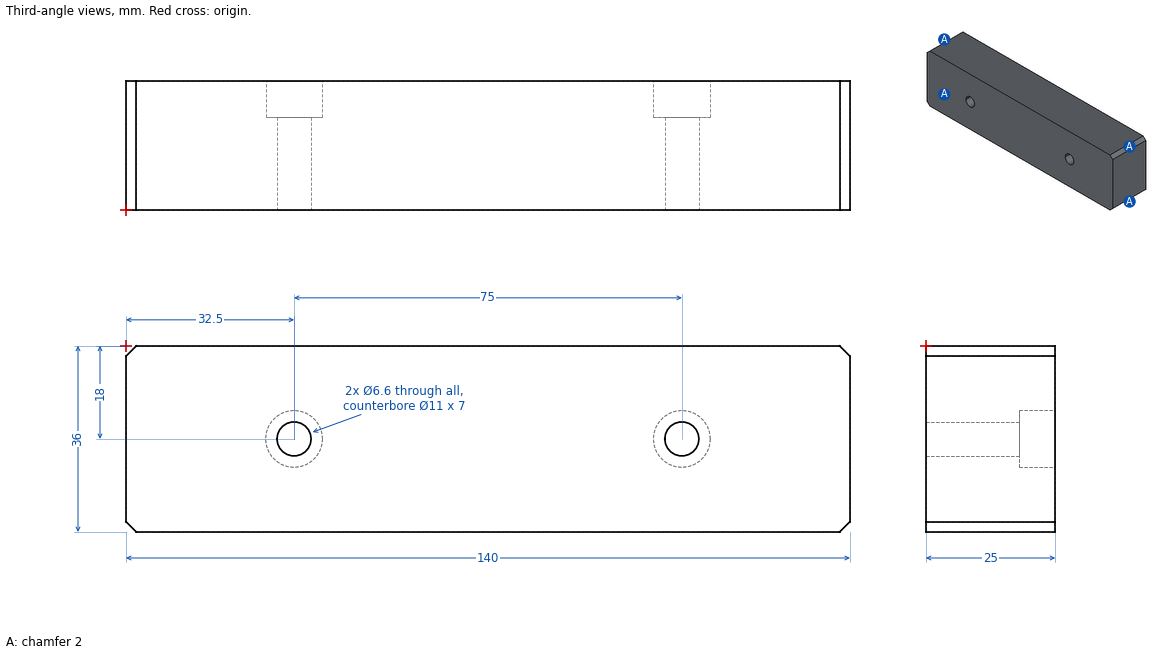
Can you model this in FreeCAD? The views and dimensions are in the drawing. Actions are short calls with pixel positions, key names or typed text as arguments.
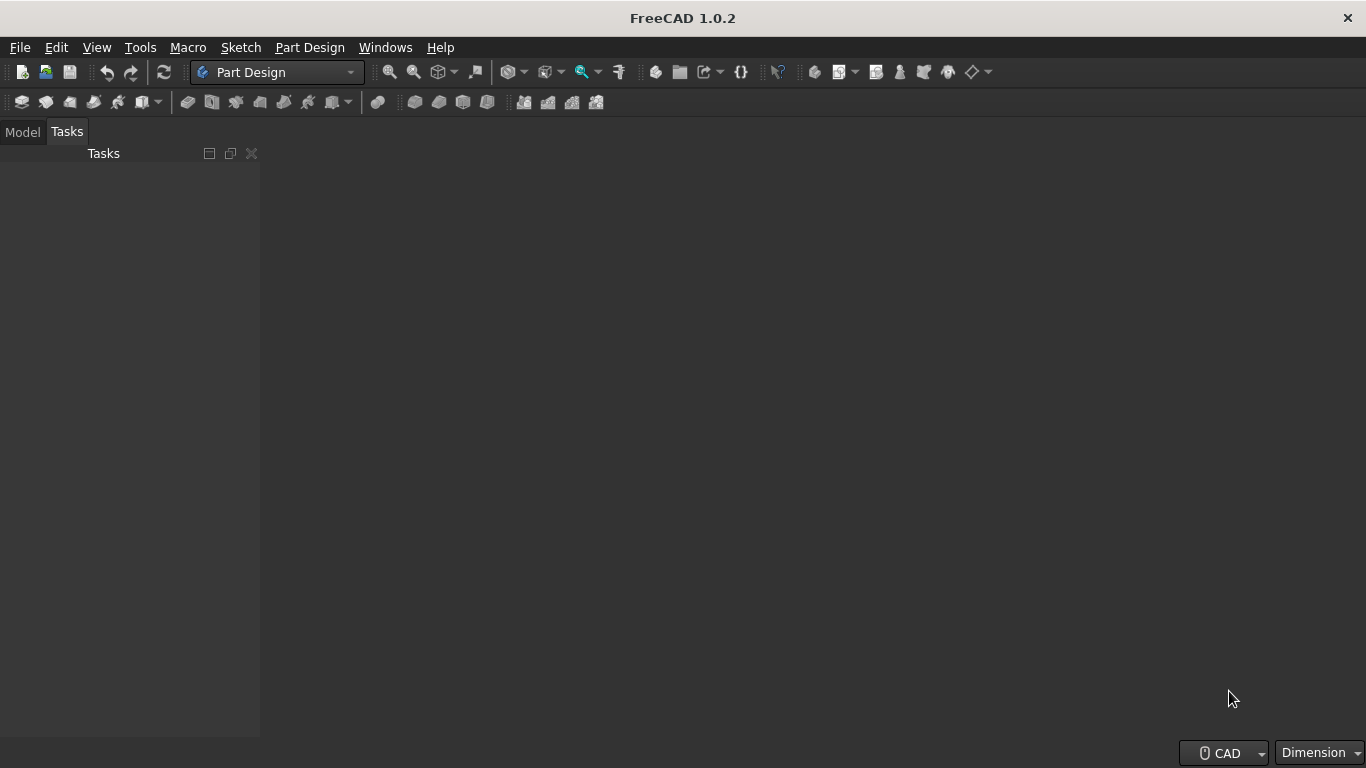
key(ctrl+n)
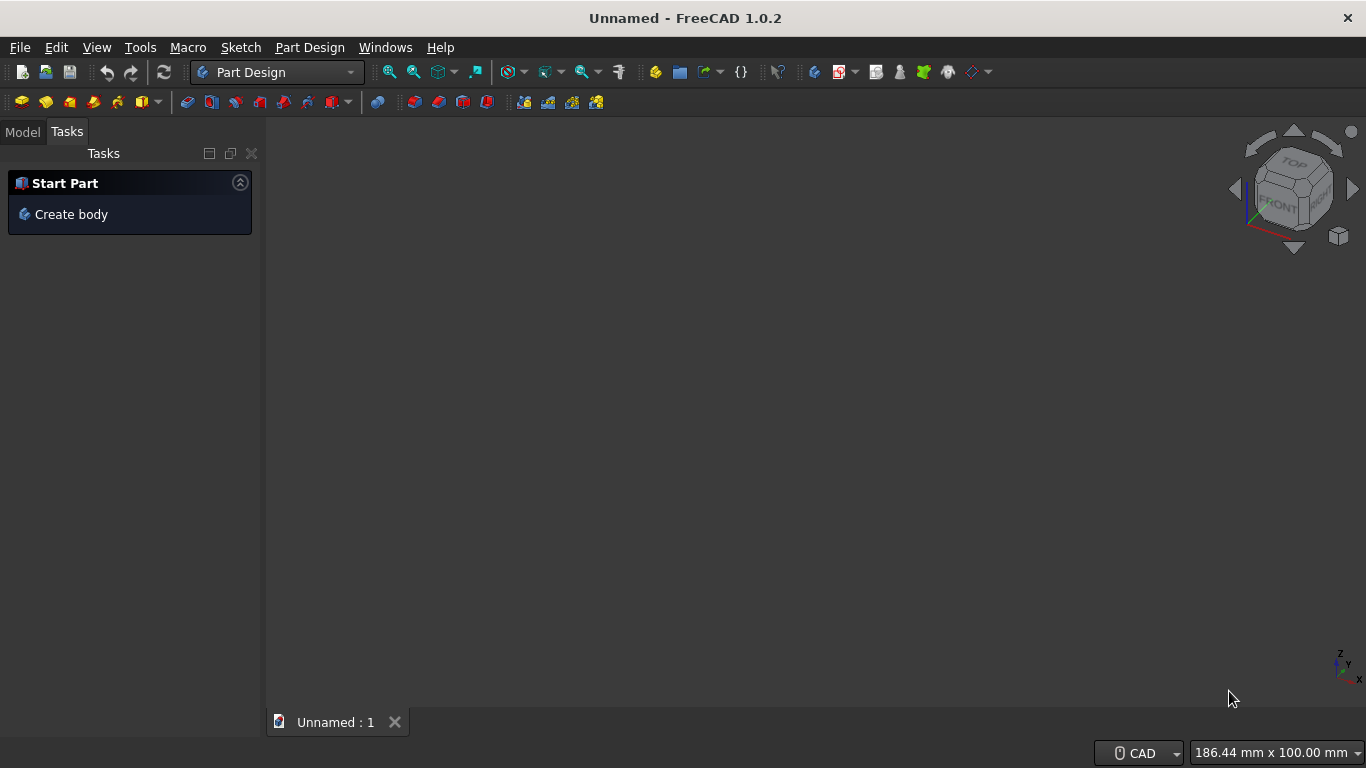
click(840, 72)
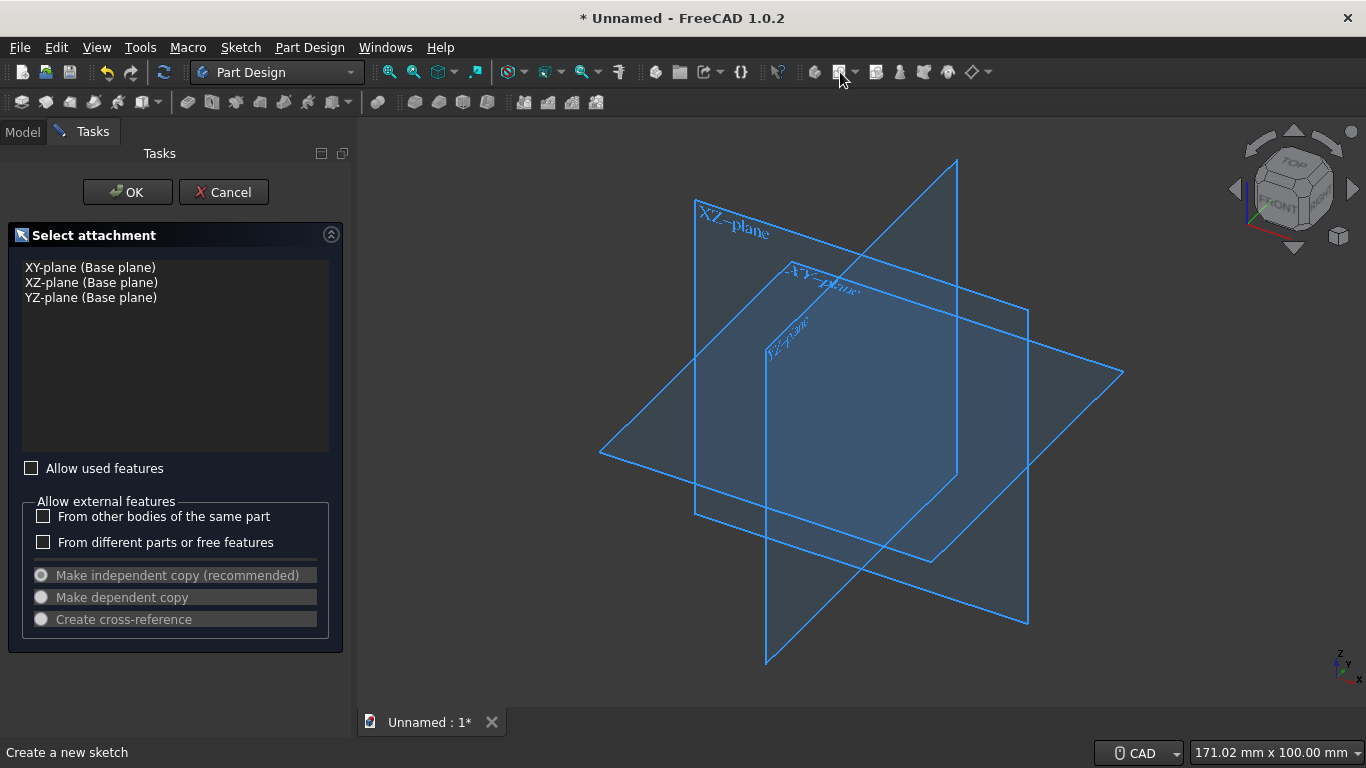
click(82, 282)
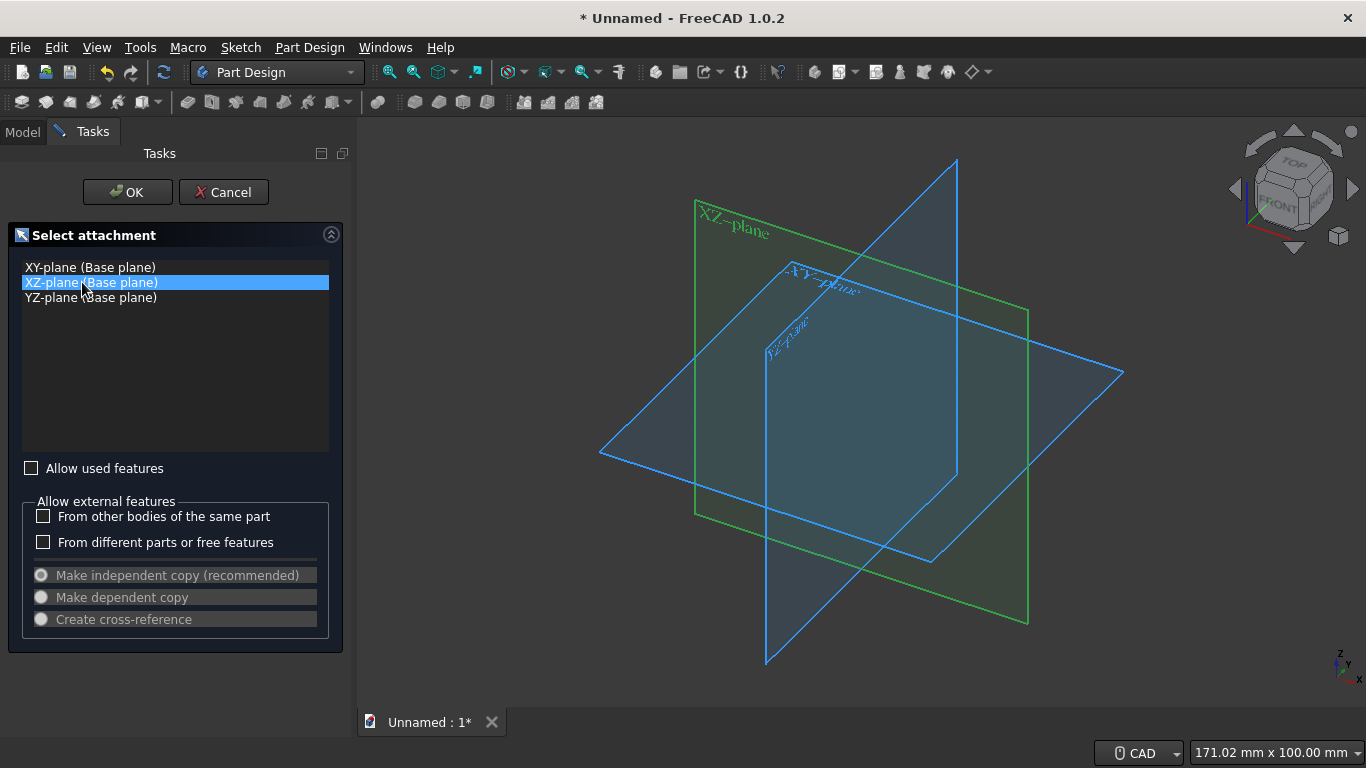
click(128, 192)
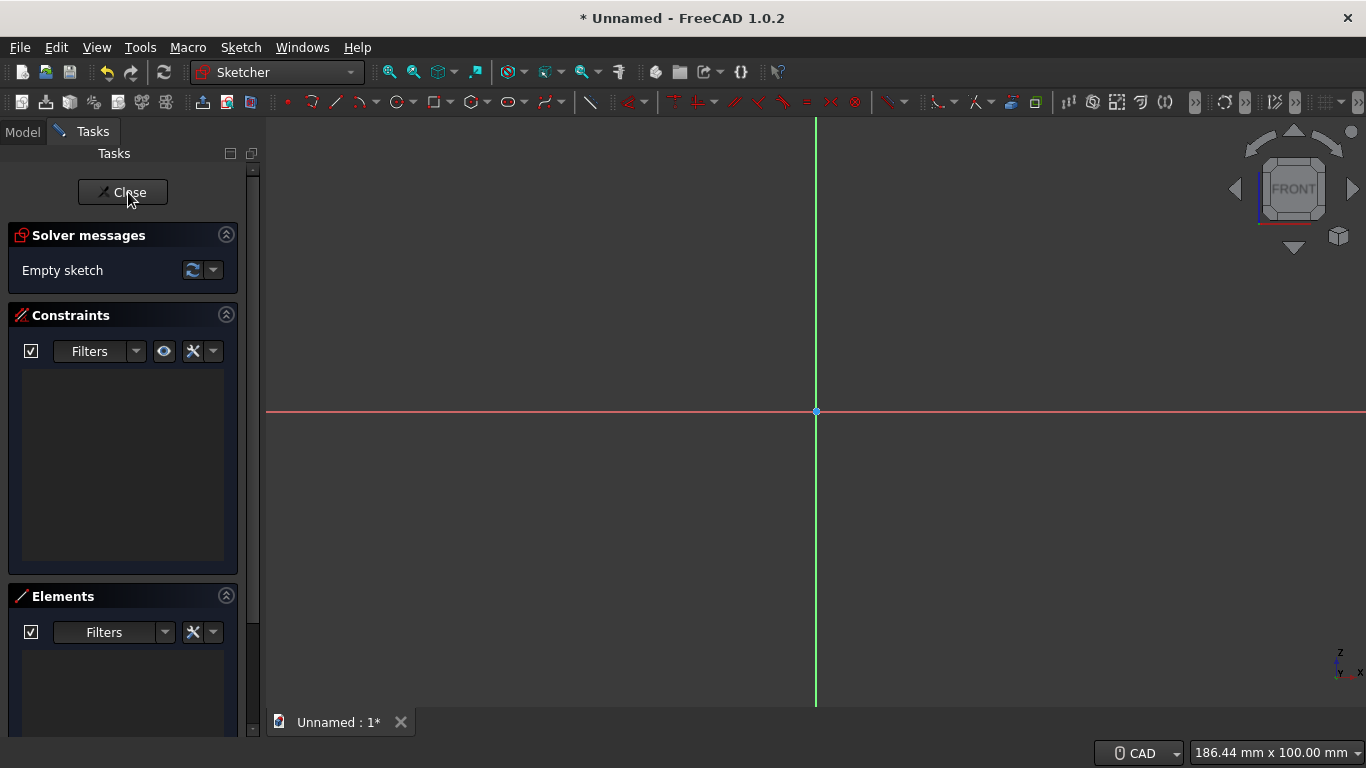
scroll(294, 283, down, 3)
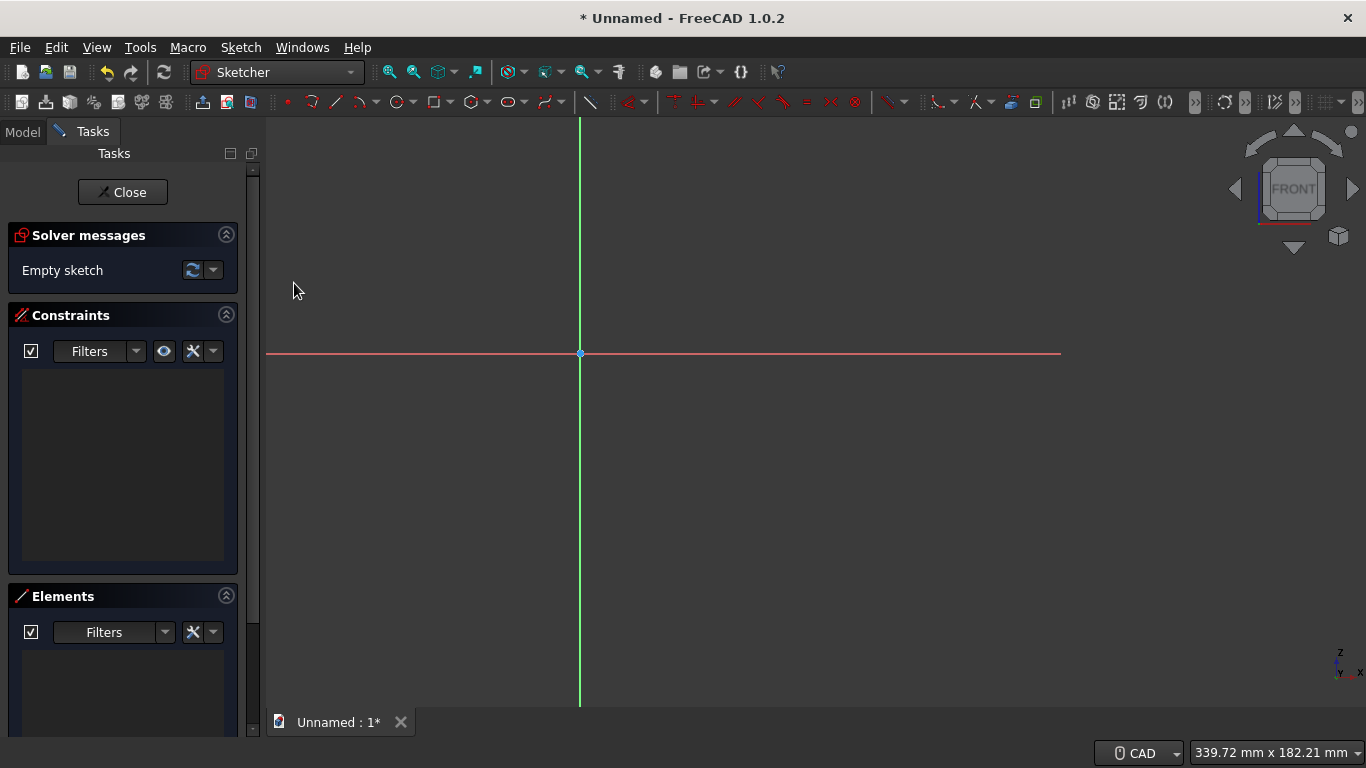
scroll(928, 413, up, 2)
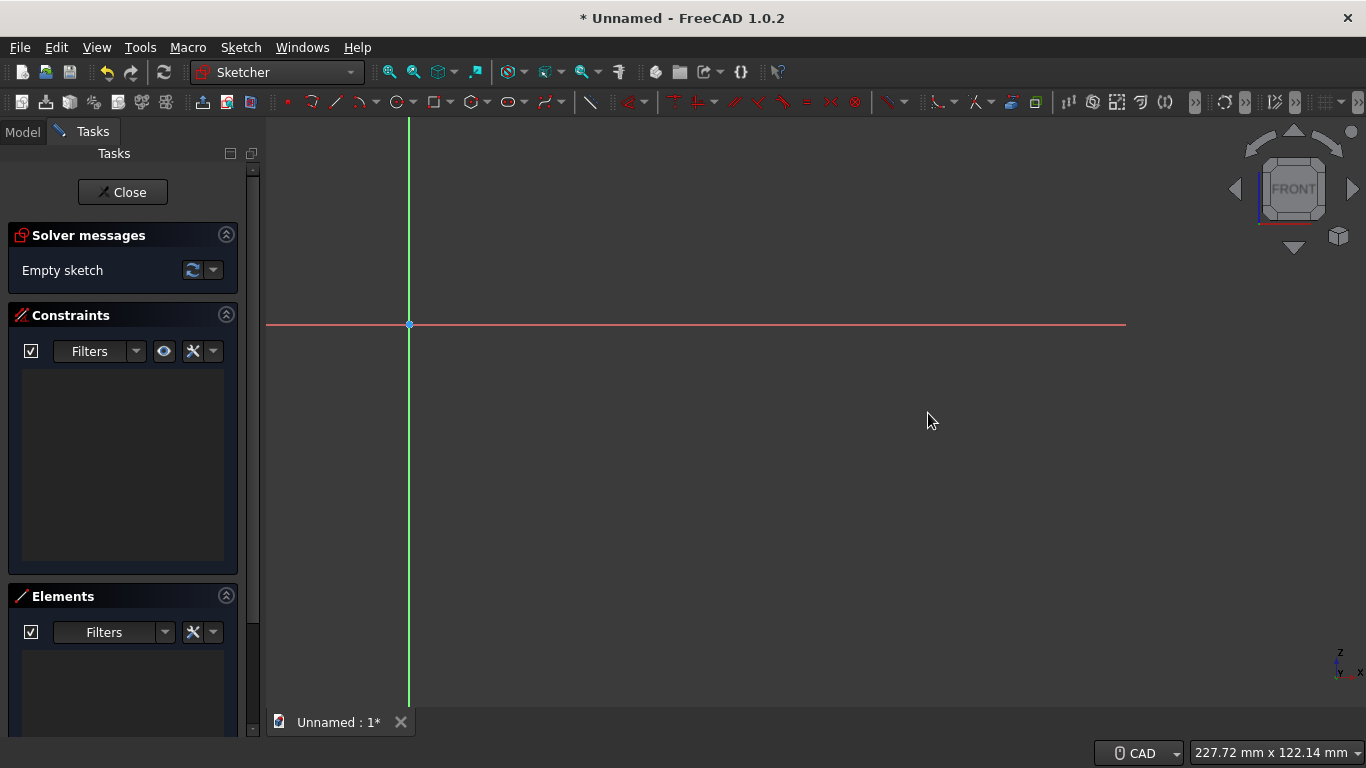
click(434, 102)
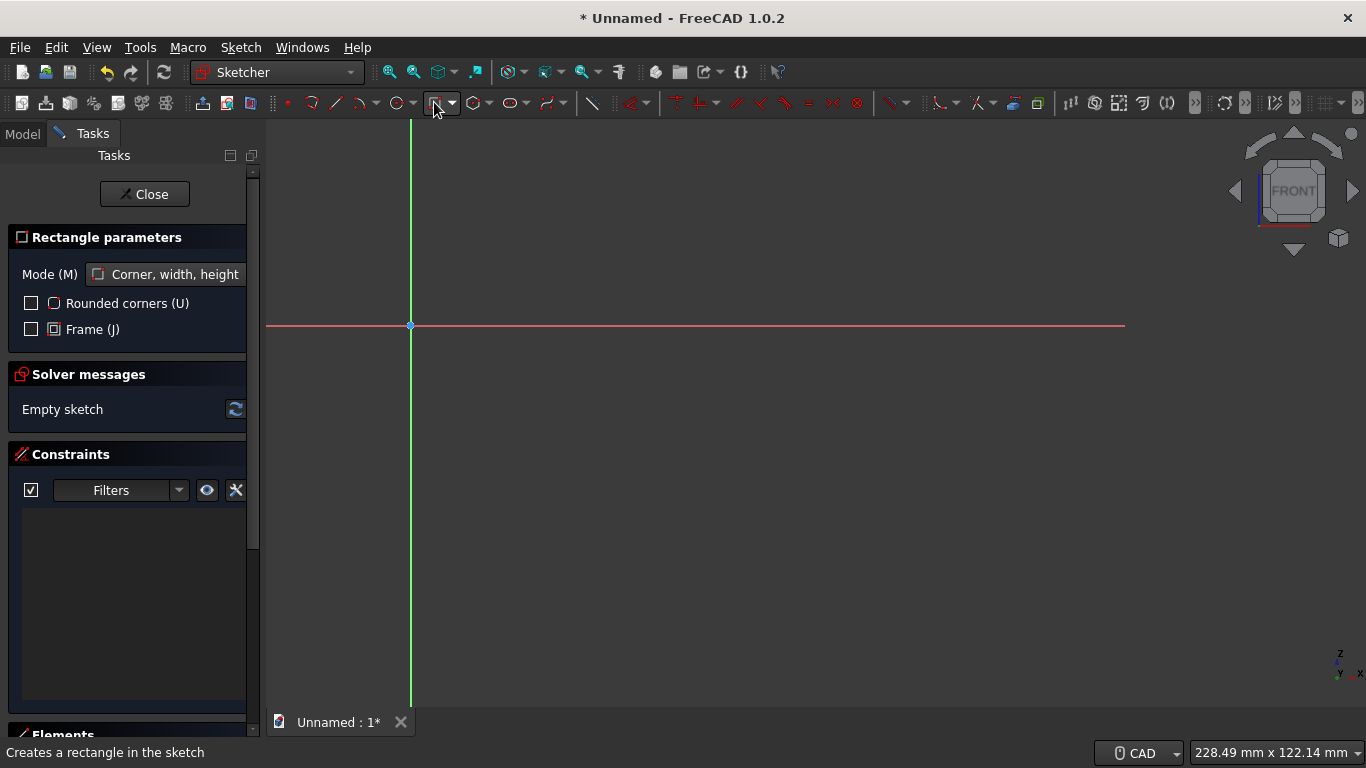
click(411, 326)
click(1085, 499)
key(Escape)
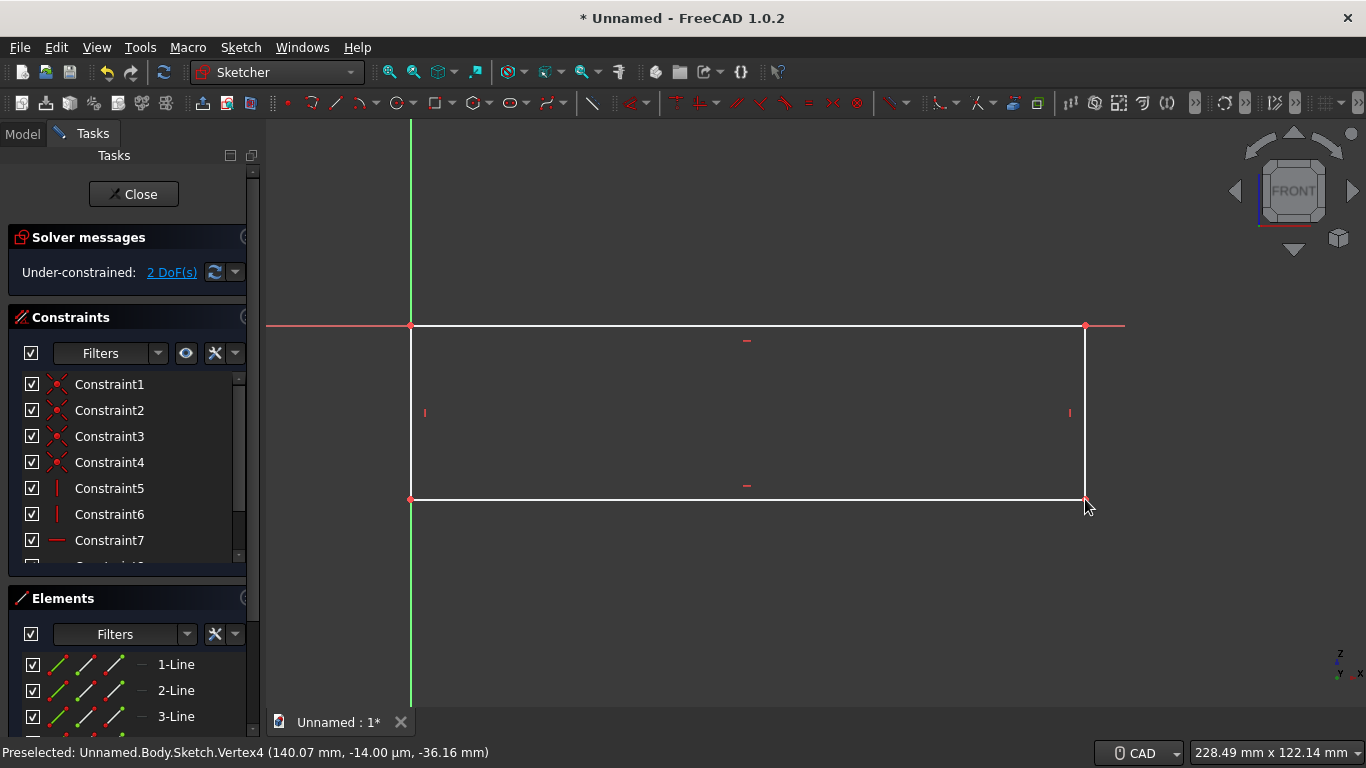
click(630, 104)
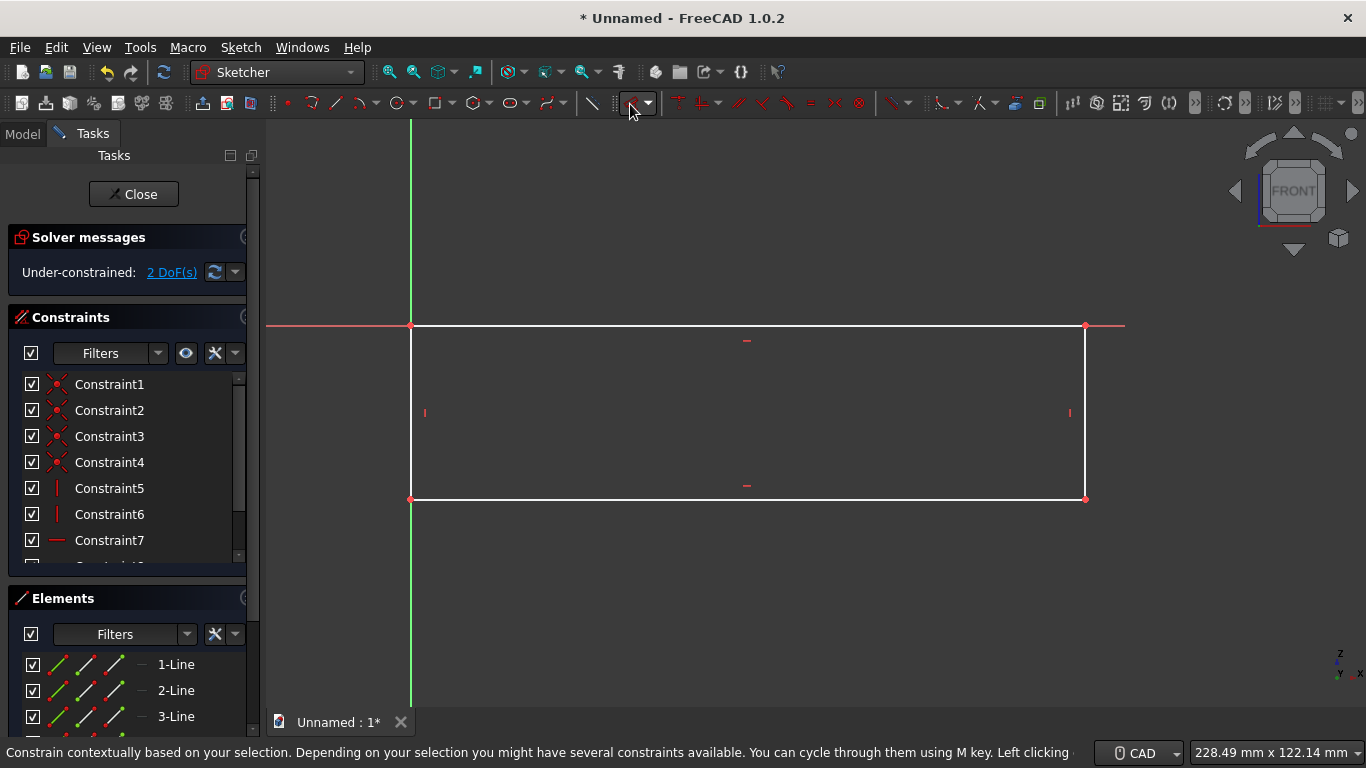
click(411, 378)
click(377, 413)